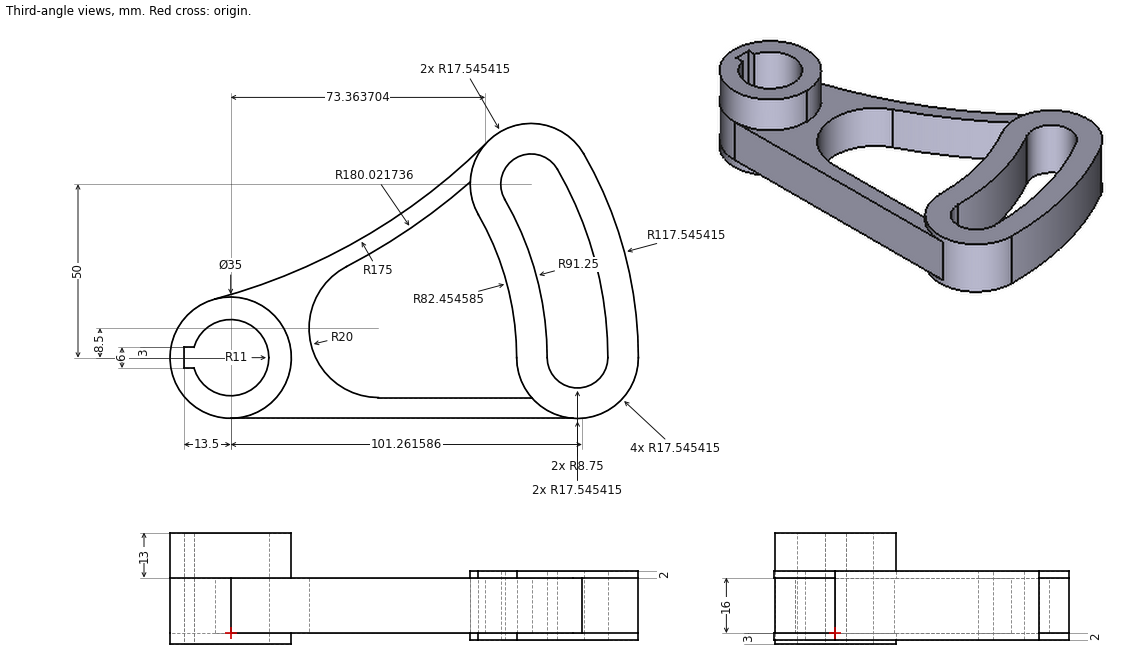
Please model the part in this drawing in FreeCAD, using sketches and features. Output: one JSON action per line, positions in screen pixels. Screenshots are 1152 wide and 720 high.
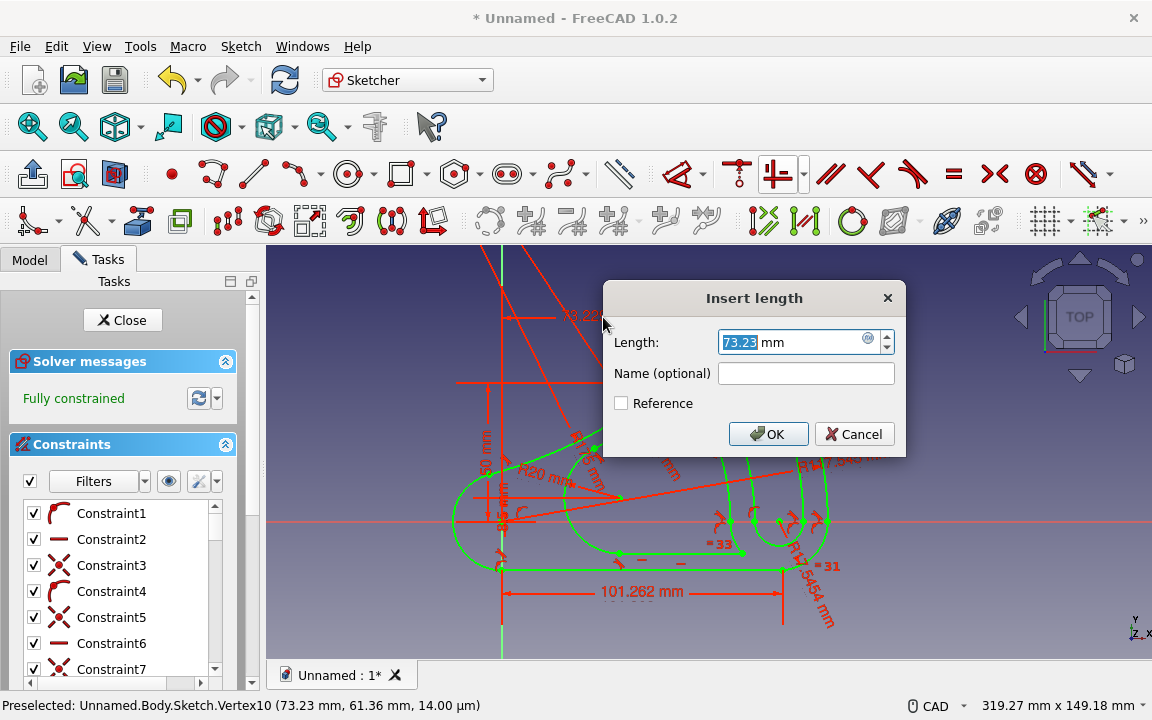
{"action": "type", "text": "73.363704"}
{"action": "key", "text": "Return"}
{"action": "key", "text": "Escape"}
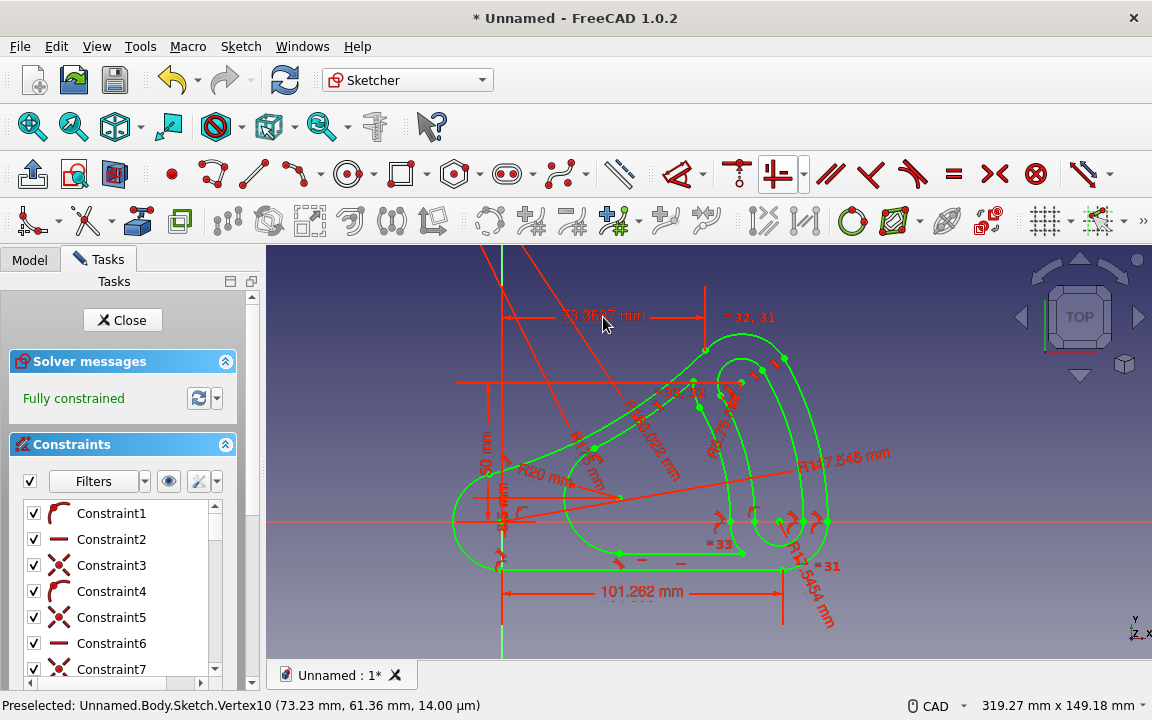
{"action": "left_click", "coordinate": [123, 320]}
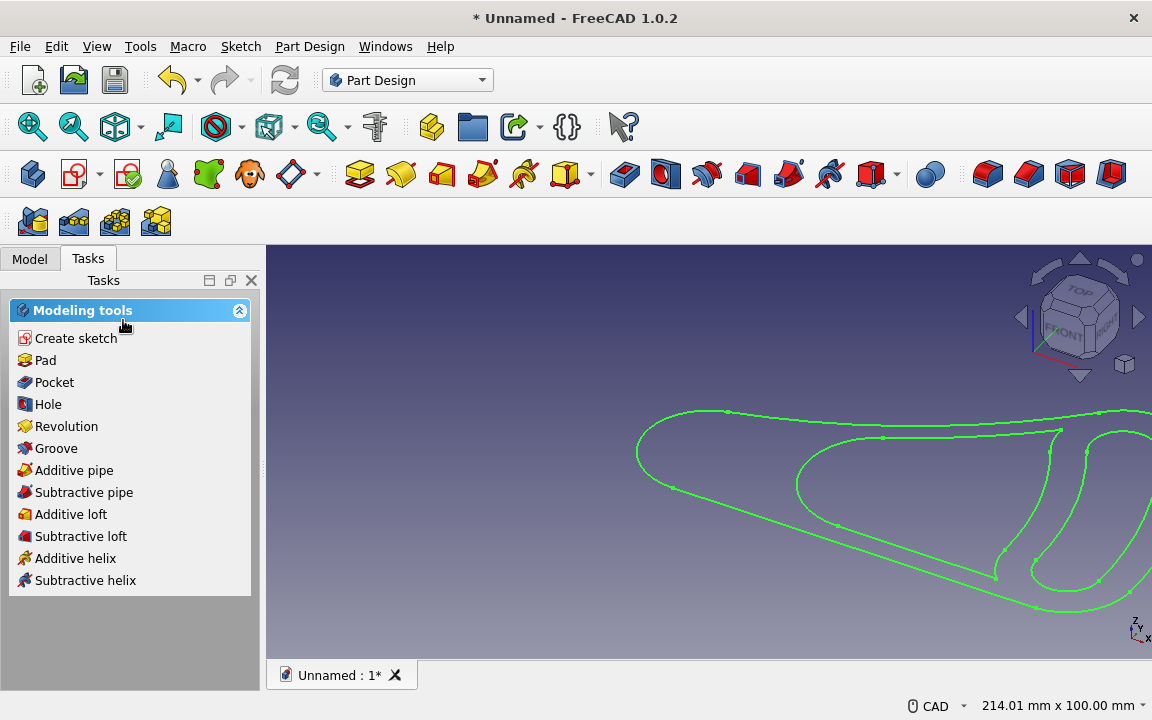
{"action": "left_click", "coordinate": [360, 174]}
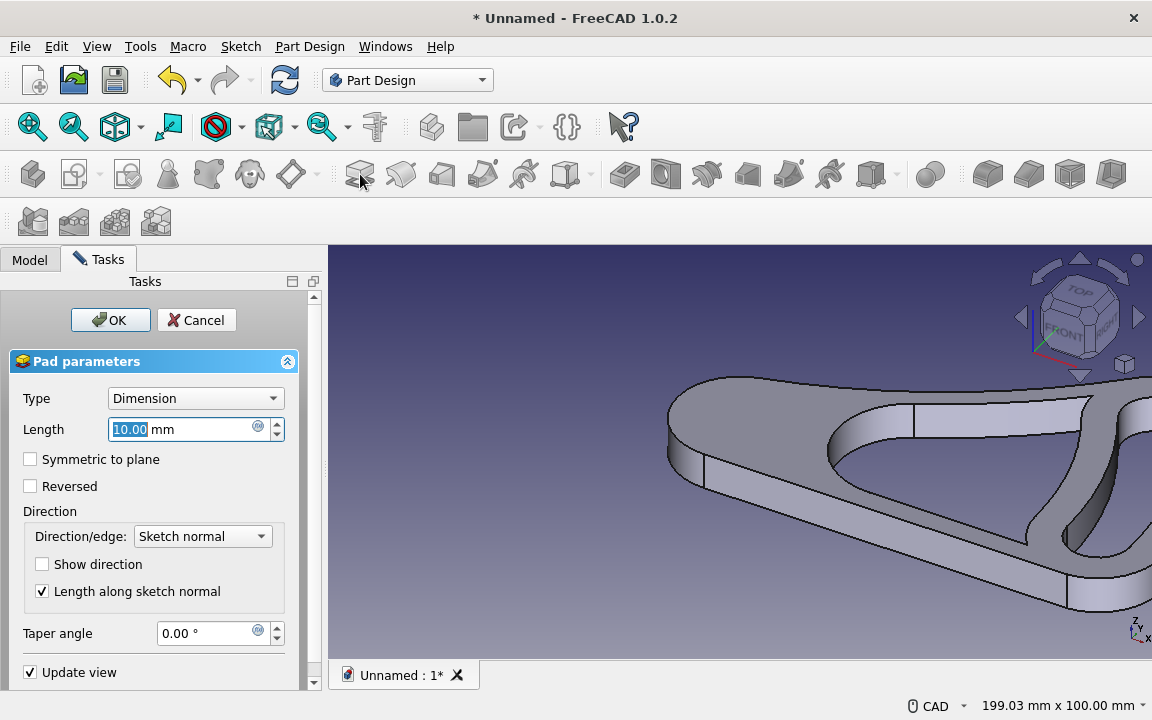
{"action": "type", "text": "16"}
{"action": "key", "text": "Tab"}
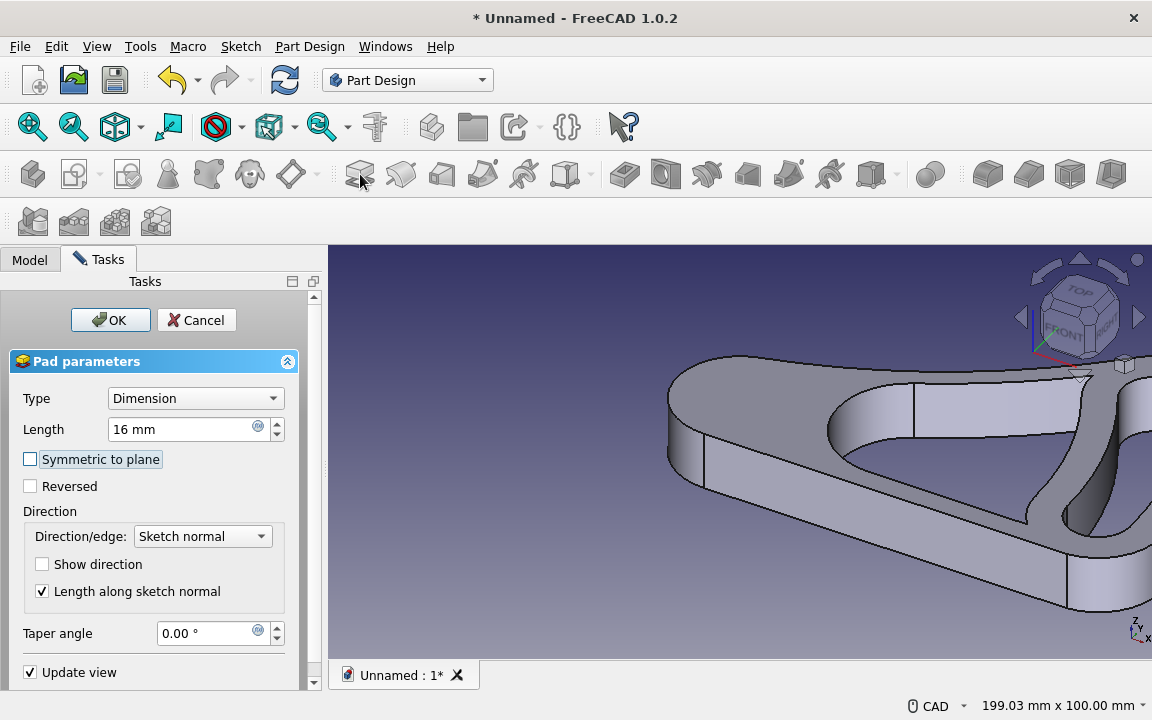
{"action": "left_click", "coordinate": [111, 320]}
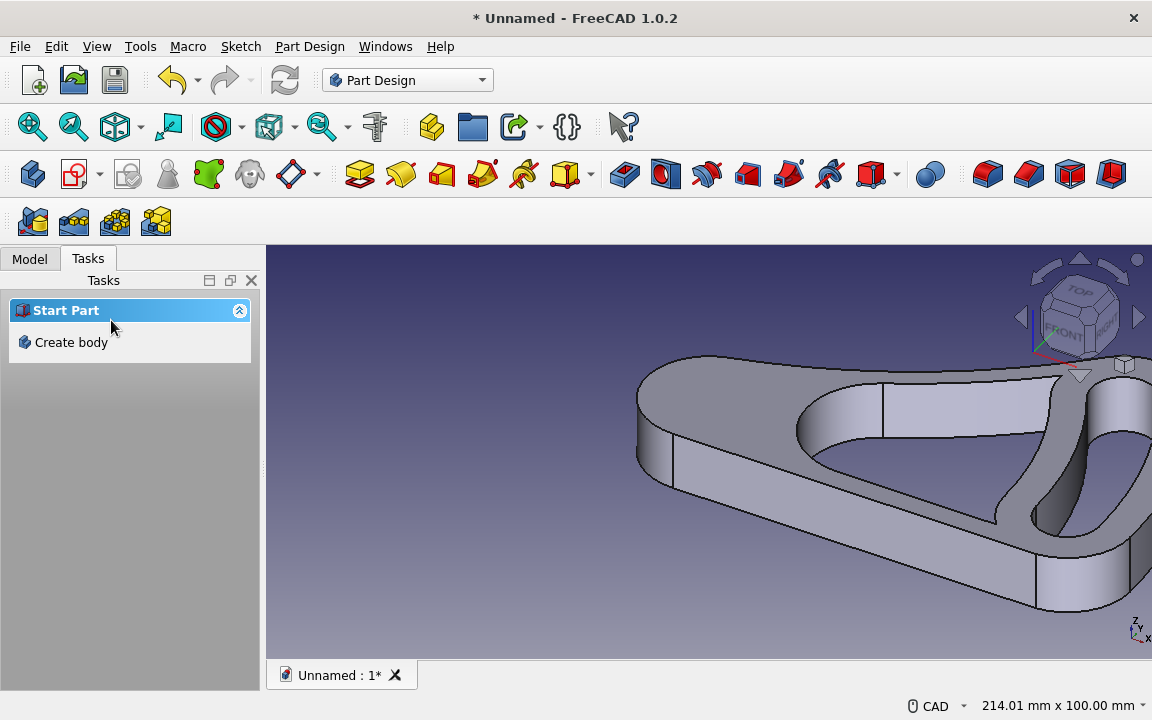
{"action": "left_click", "coordinate": [33, 128]}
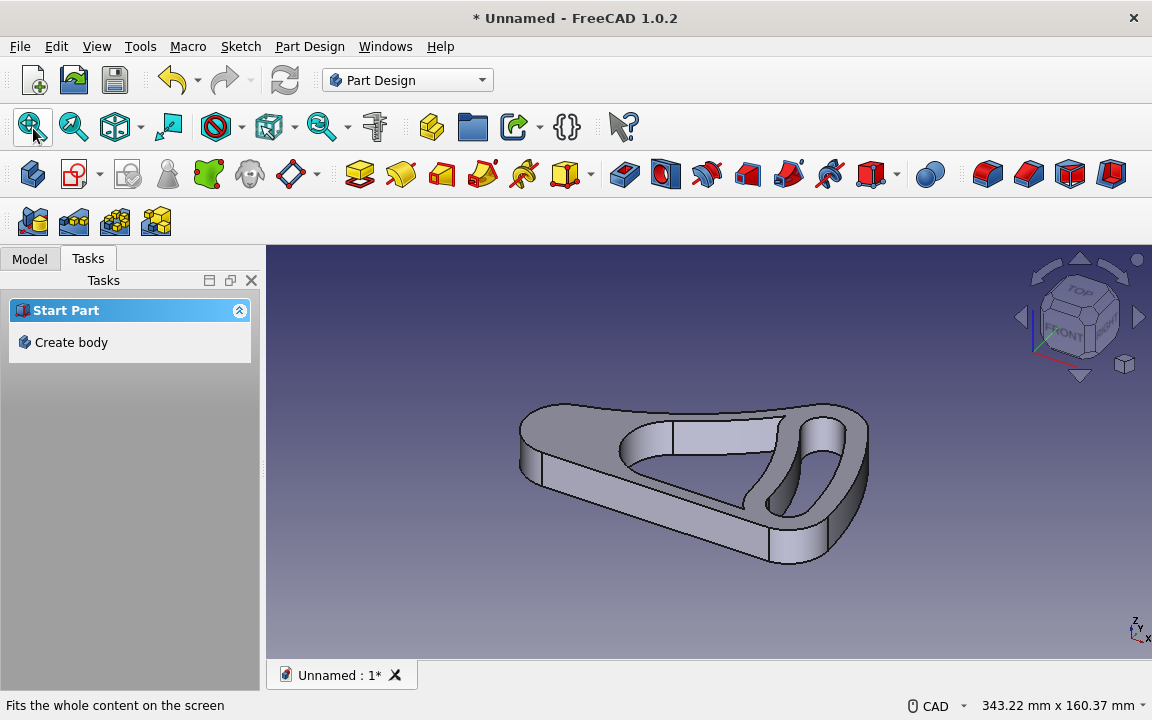
{"action": "left_click", "coordinate": [591, 437]}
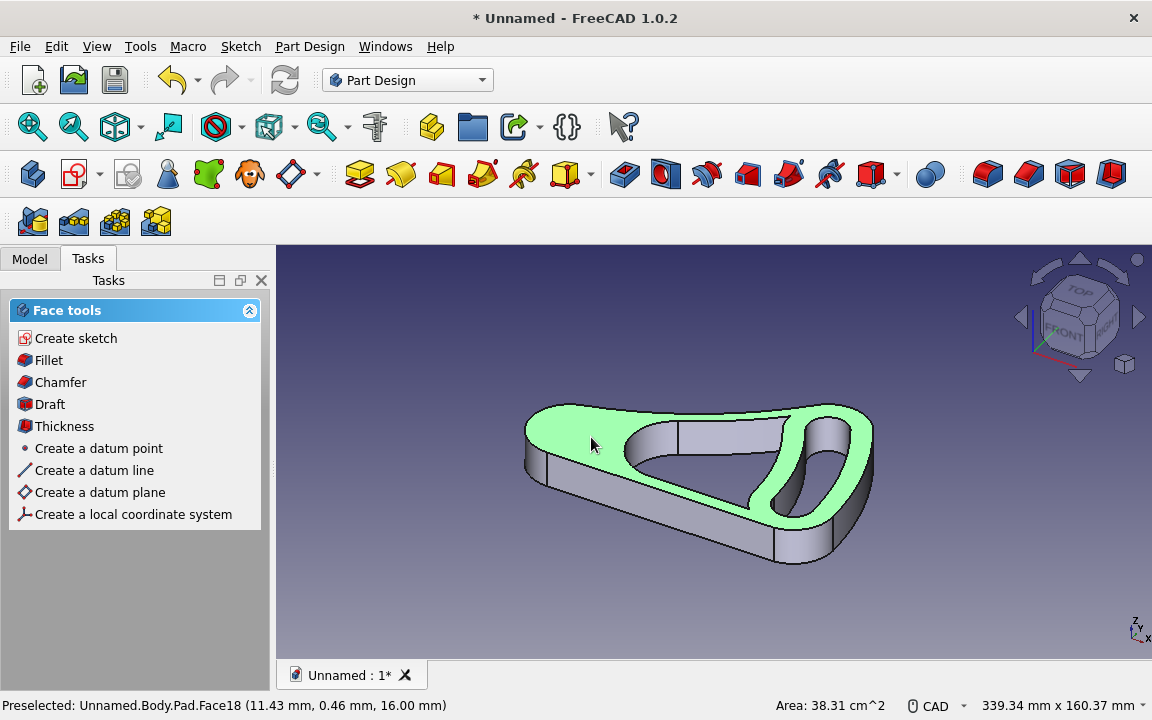
{"action": "left_click", "coordinate": [74, 174]}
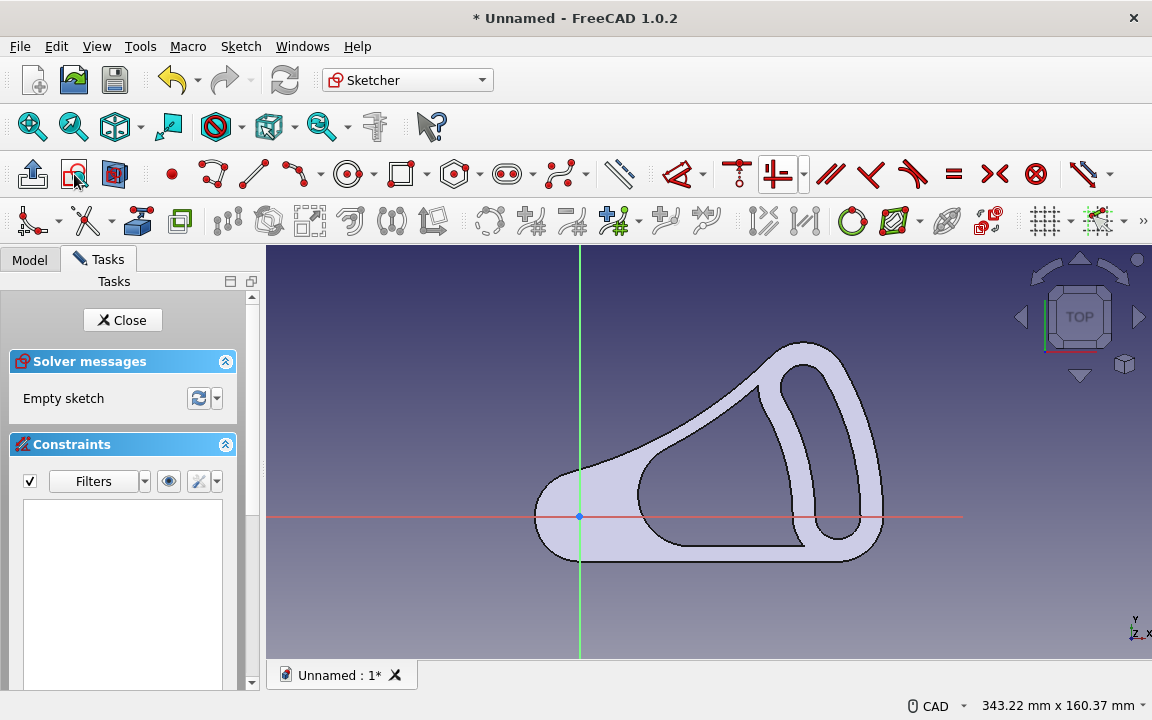
{"action": "scroll", "coordinate": [545, 554], "scroll_direction": "up", "scroll_amount": 5}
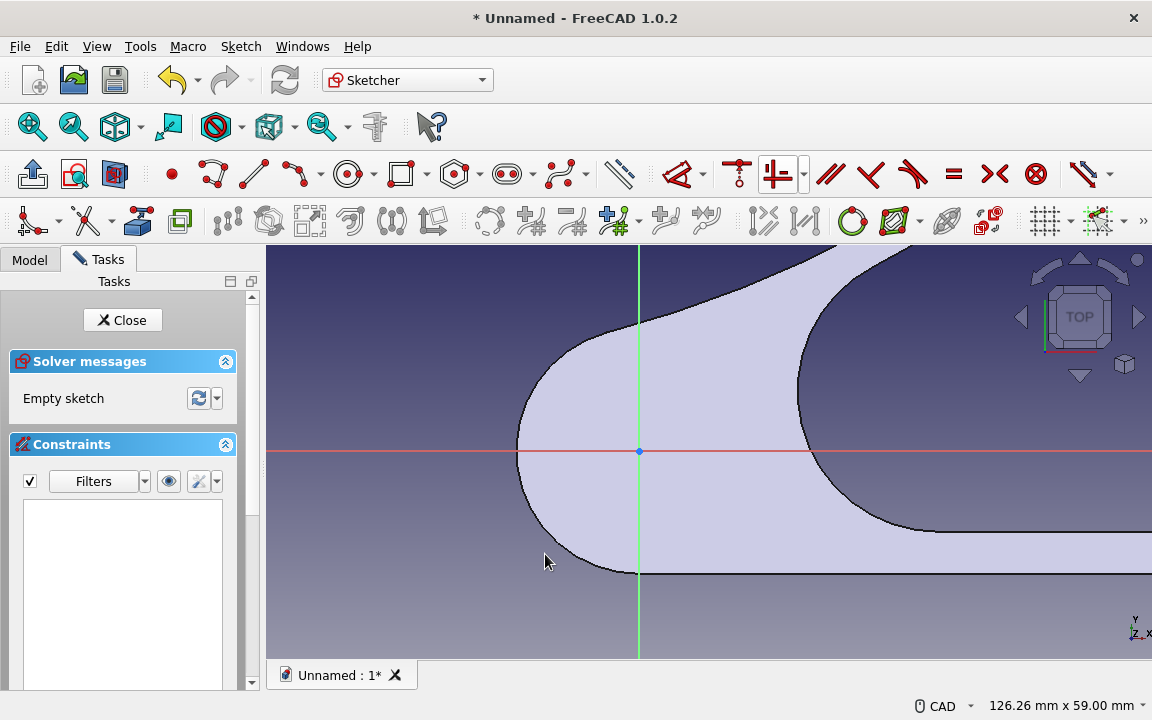
{"action": "left_click", "coordinate": [348, 174]}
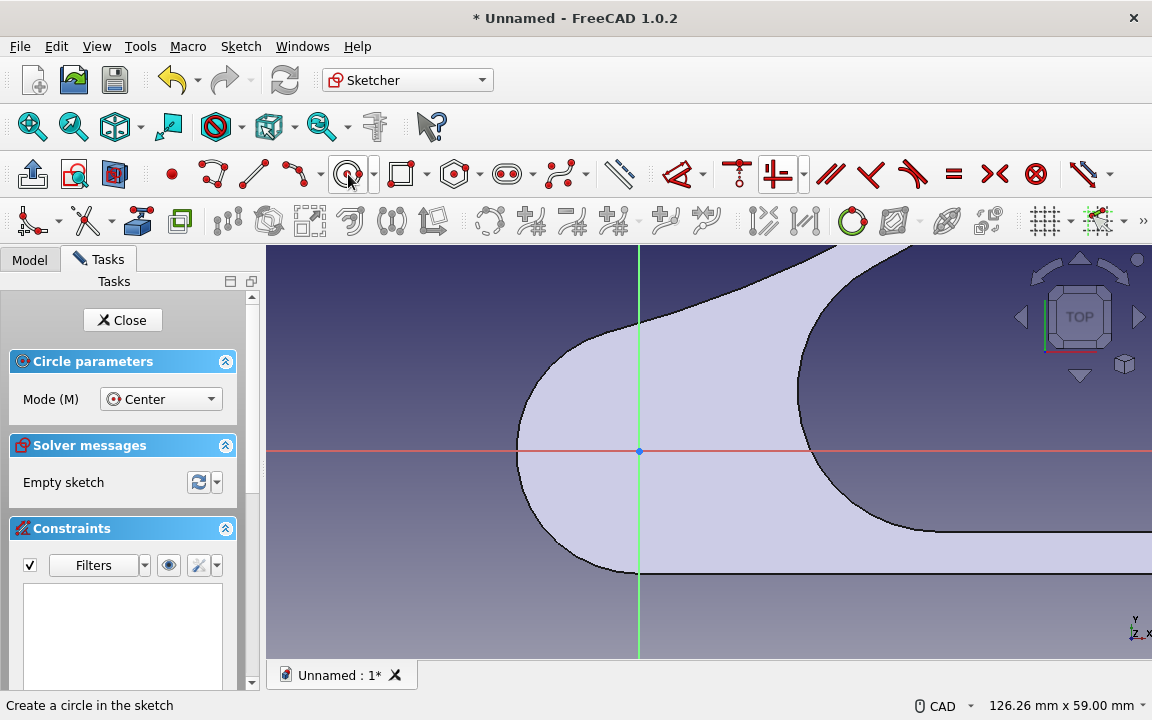
{"action": "left_click", "coordinate": [639, 451]}
{"action": "left_click", "coordinate": [726, 364]}
{"action": "key", "text": "Escape"}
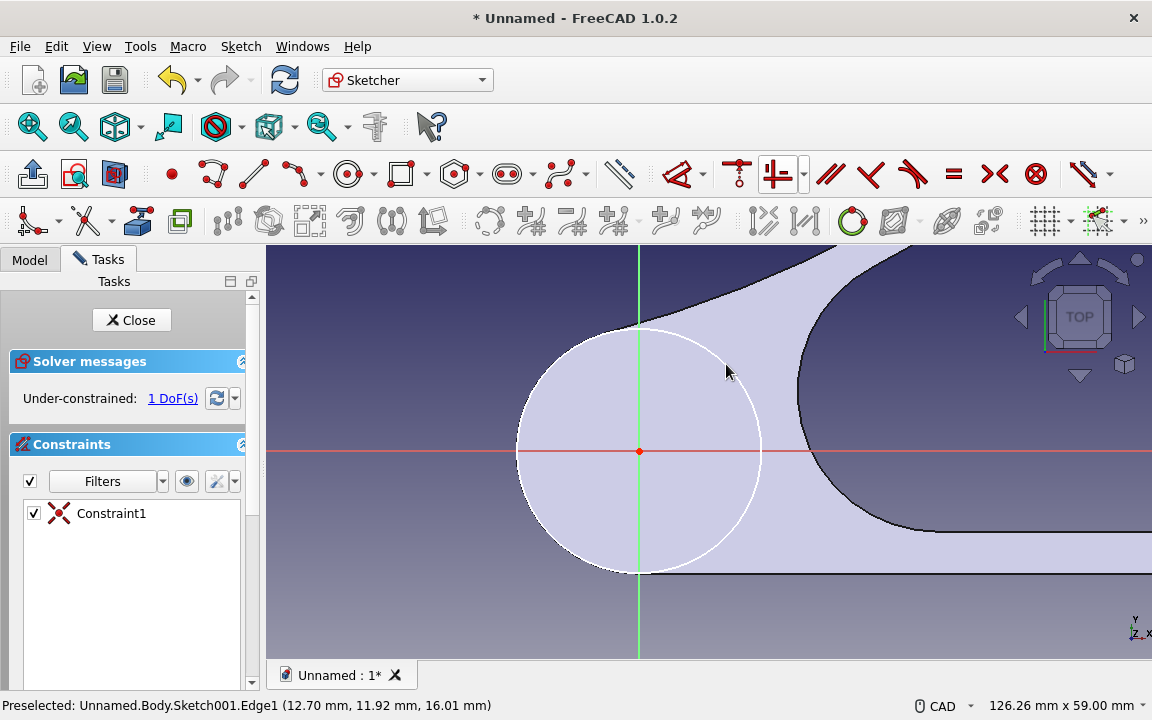
{"action": "left_click", "coordinate": [676, 174]}